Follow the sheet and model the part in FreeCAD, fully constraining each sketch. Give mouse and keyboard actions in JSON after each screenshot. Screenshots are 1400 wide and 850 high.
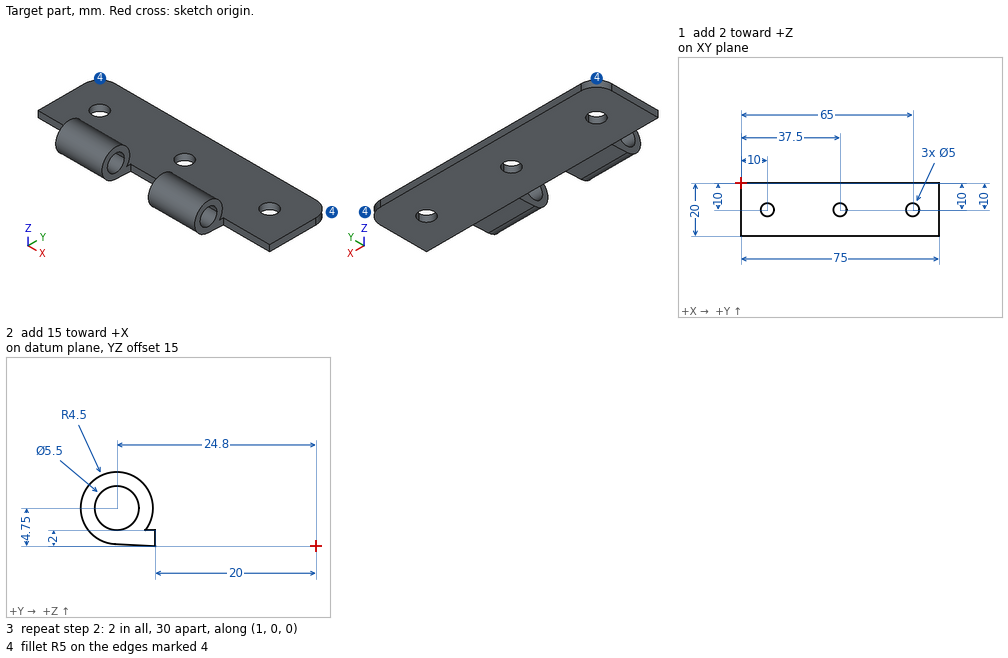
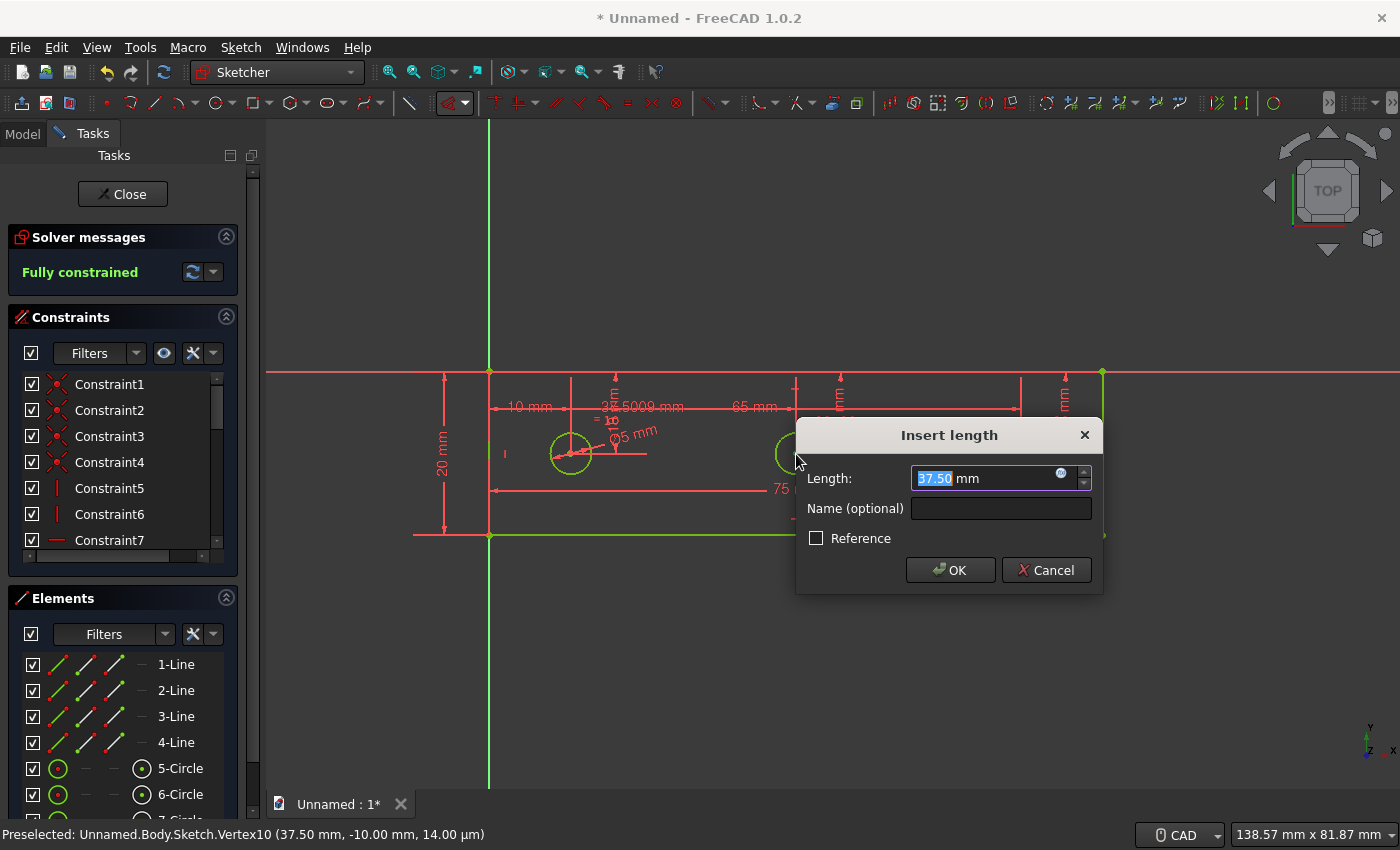
{"action": "type", "text": "37.5"}
{"action": "key", "text": "Return"}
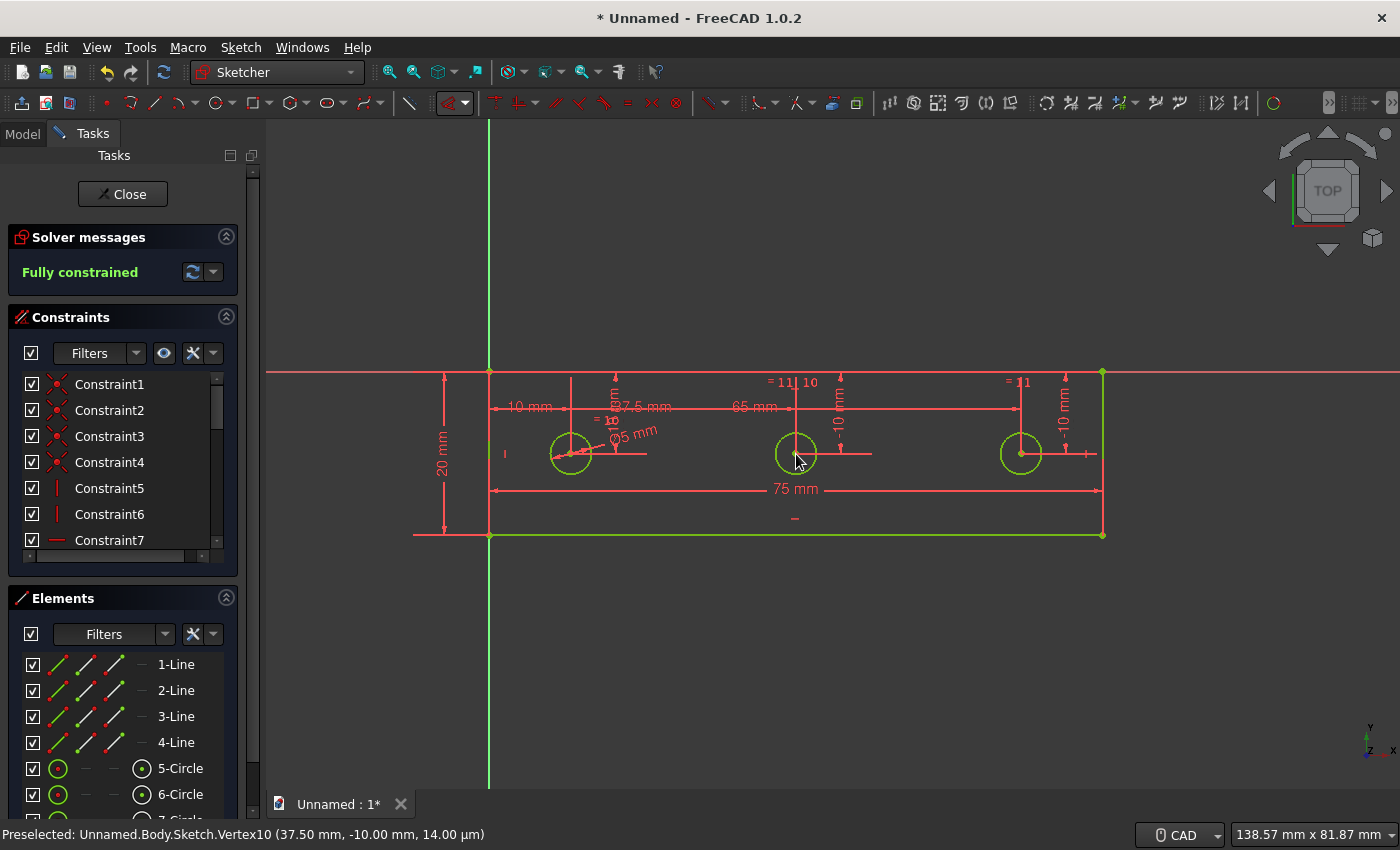
{"action": "left_click", "coordinate": [123, 194]}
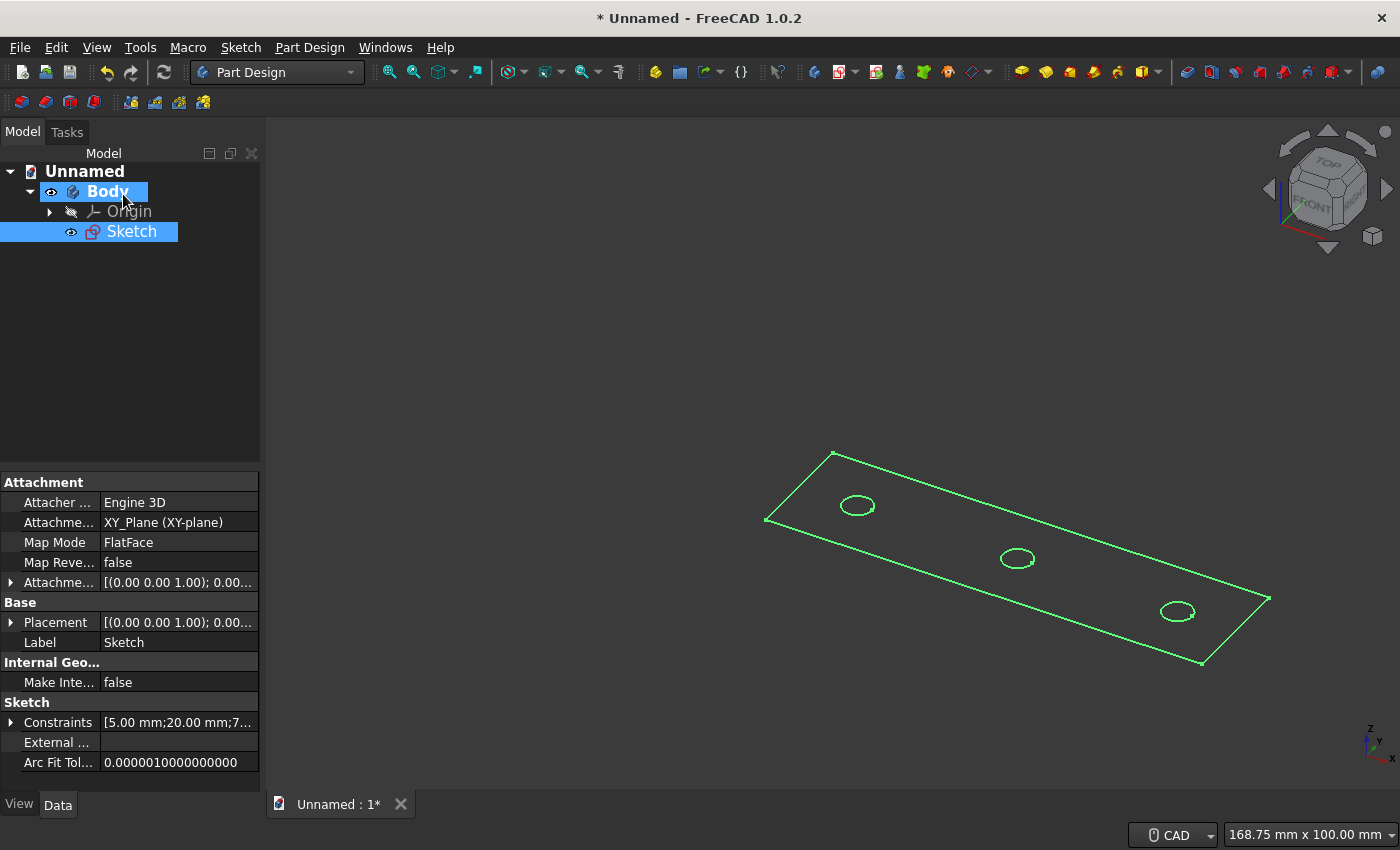
{"action": "left_click", "coordinate": [1022, 72]}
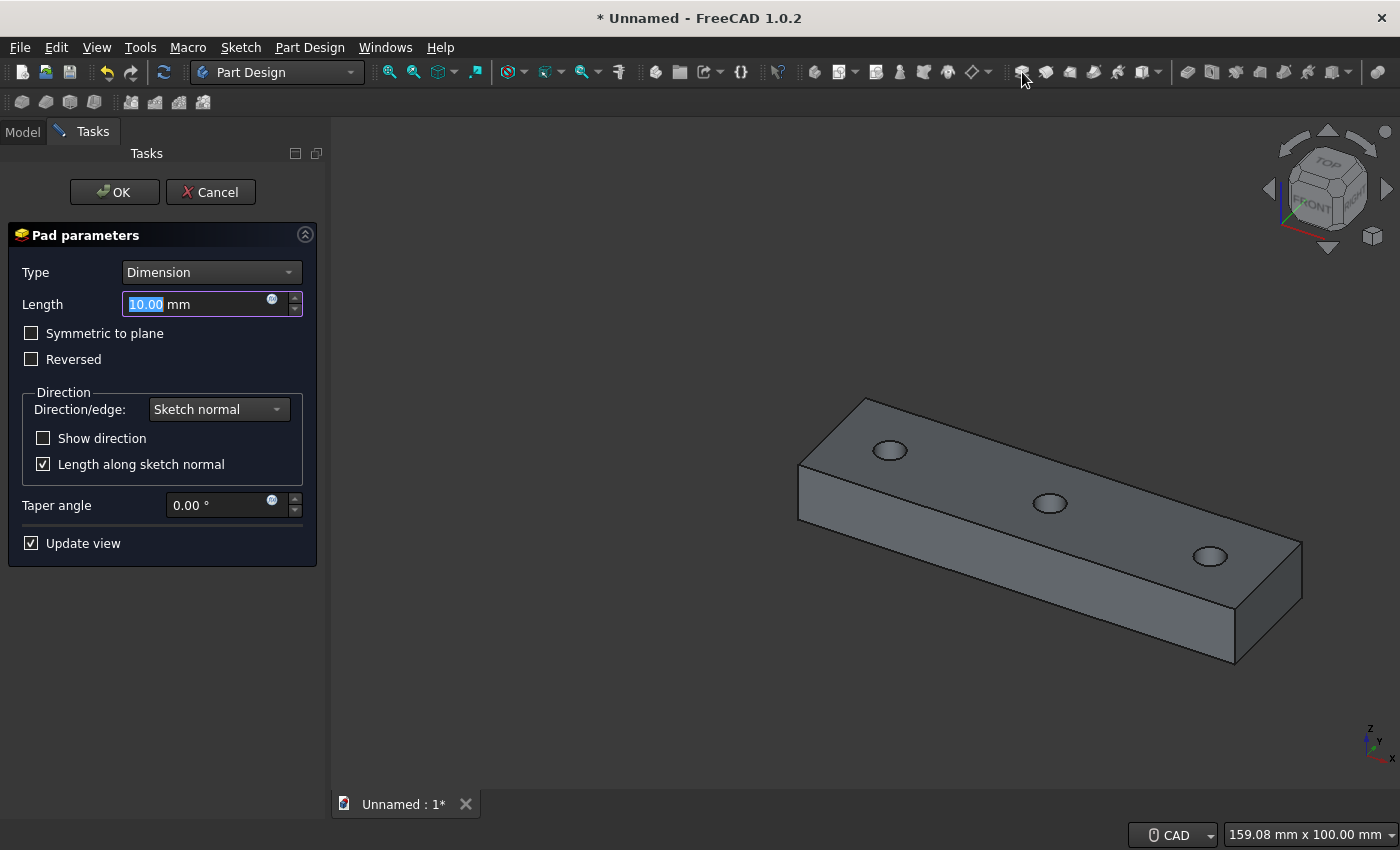
{"action": "type", "text": "2"}
{"action": "key", "text": "Tab"}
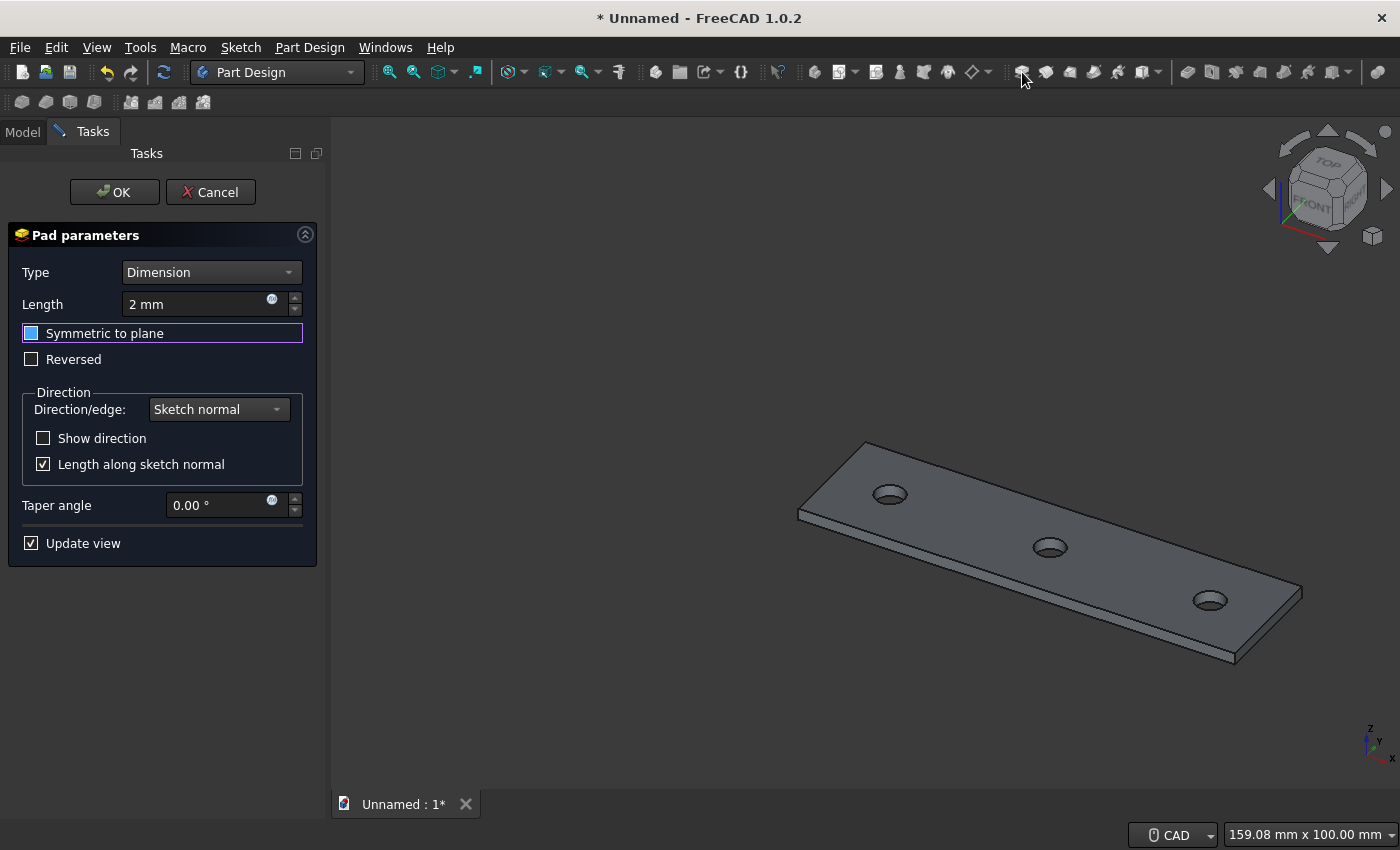
{"action": "left_click", "coordinate": [115, 192]}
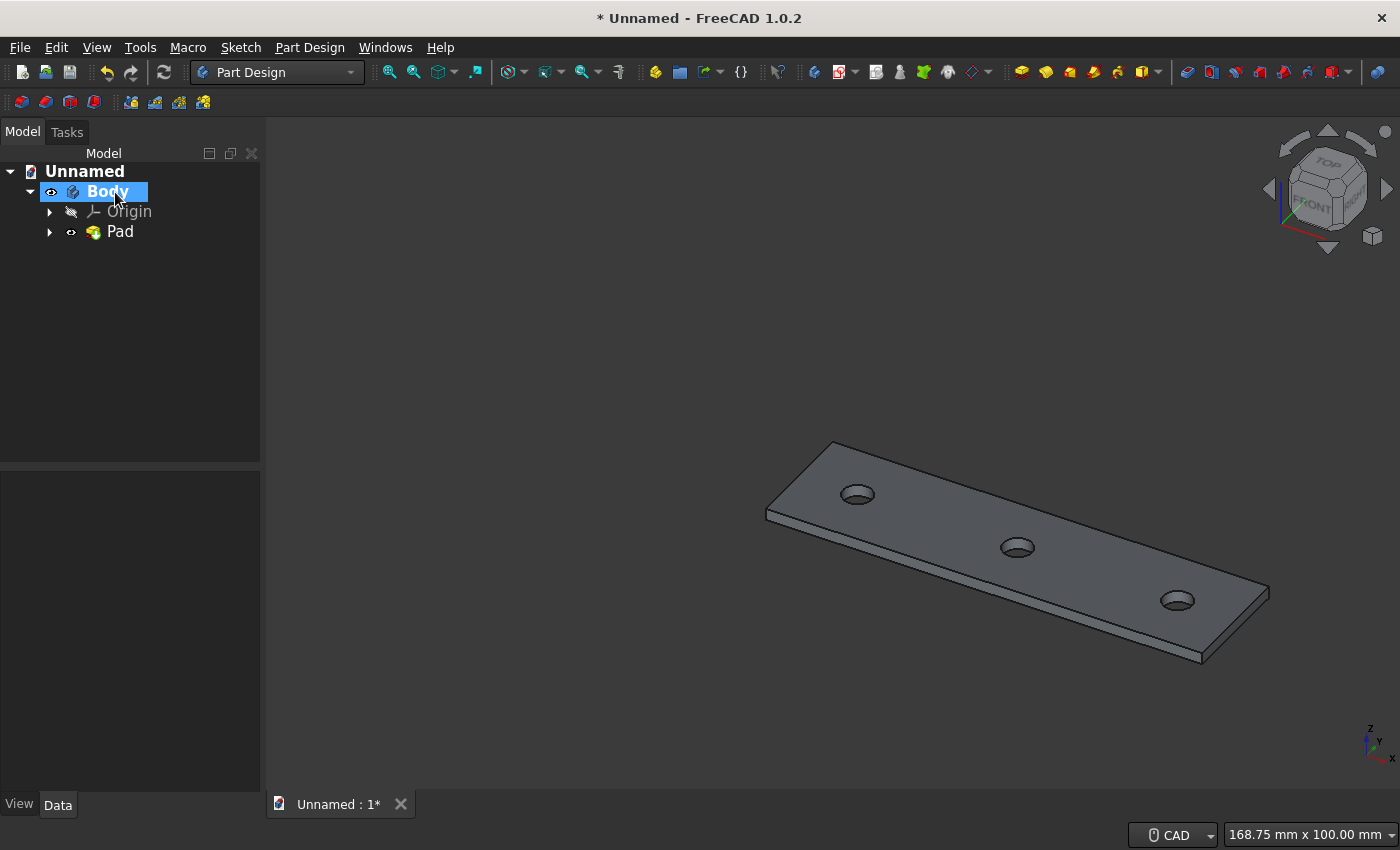
{"action": "key", "text": "v f"}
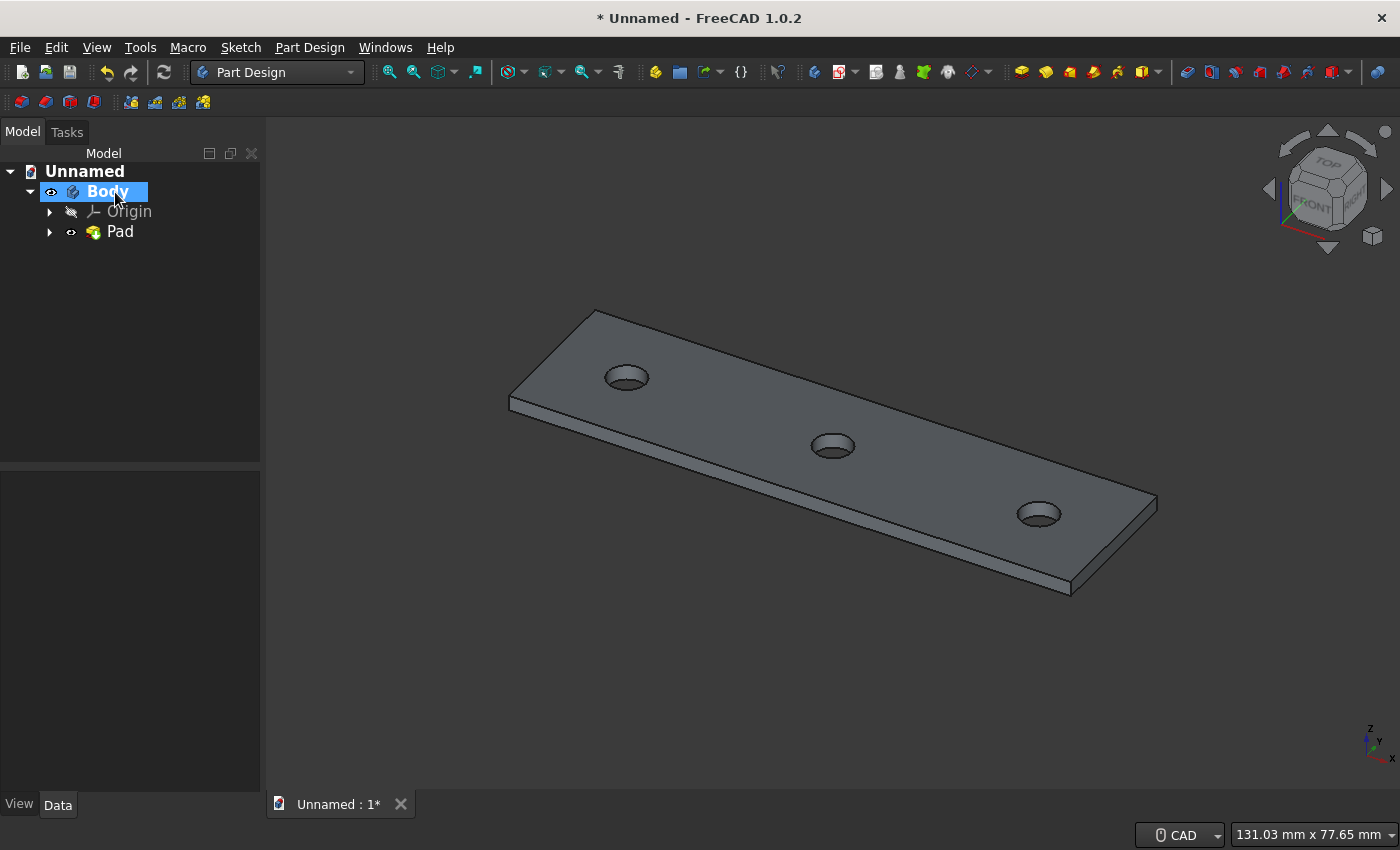
{"action": "left_click", "coordinate": [50, 212]}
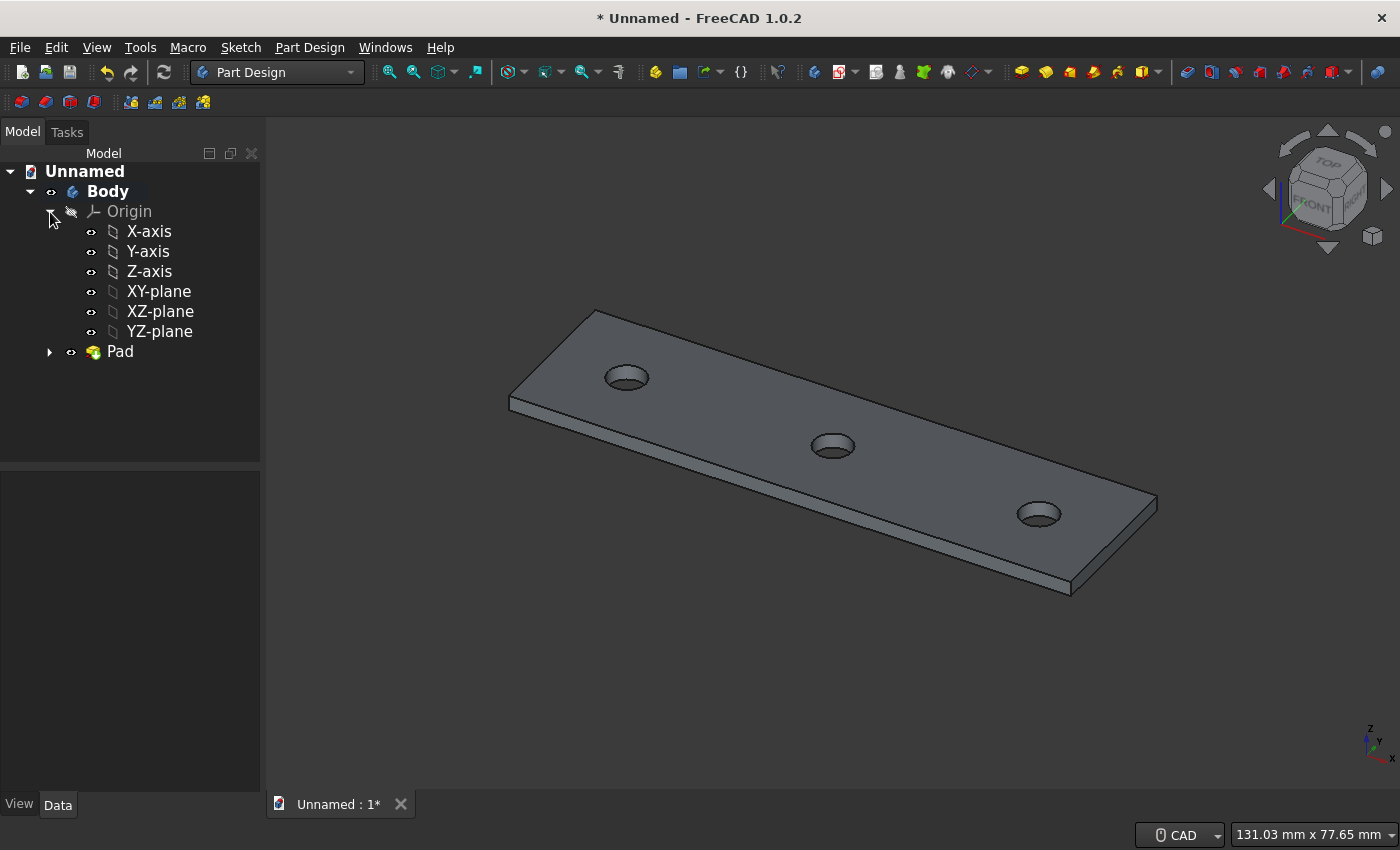
{"action": "left_click", "coordinate": [136, 332]}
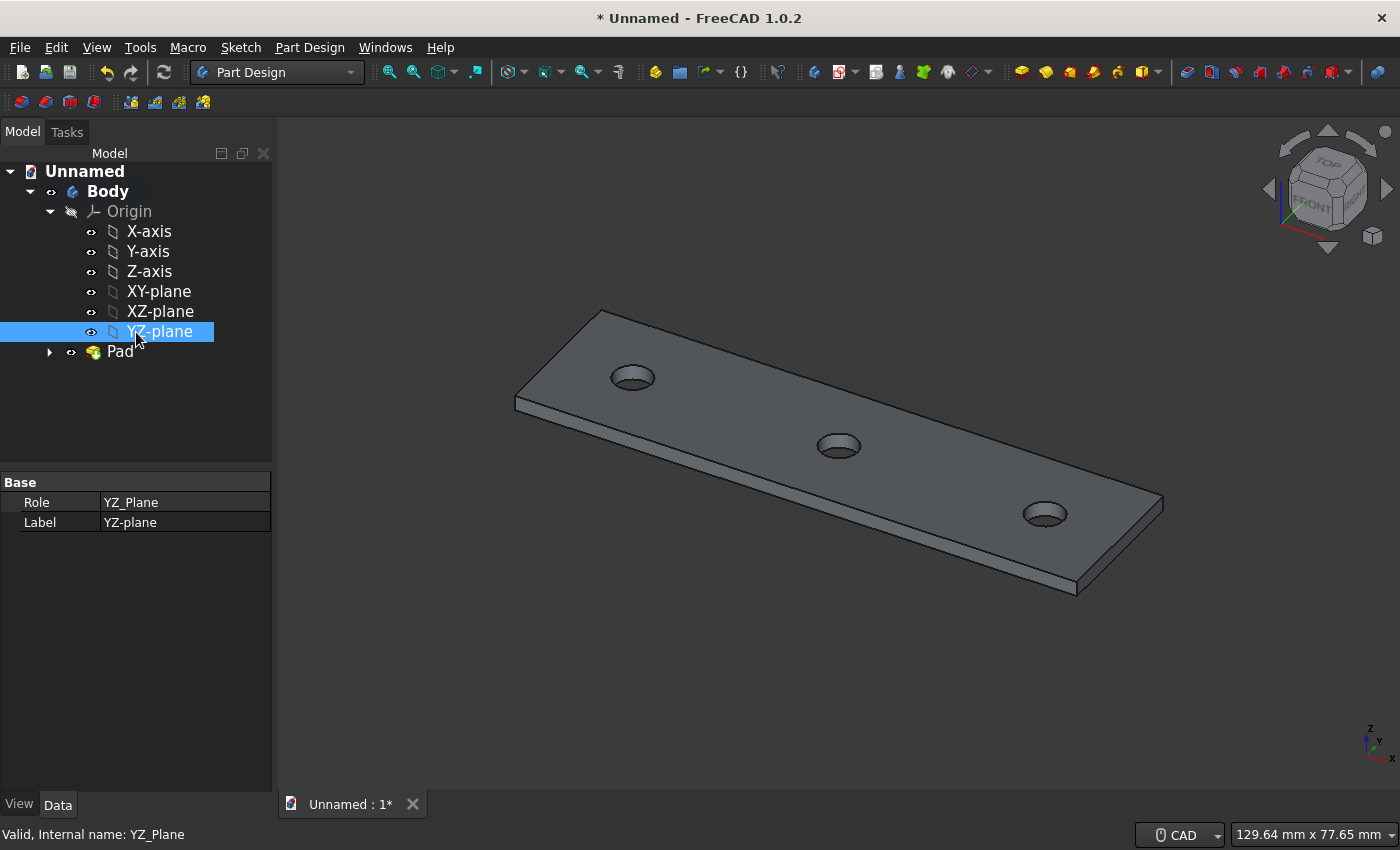
{"action": "left_click", "coordinate": [972, 72]}